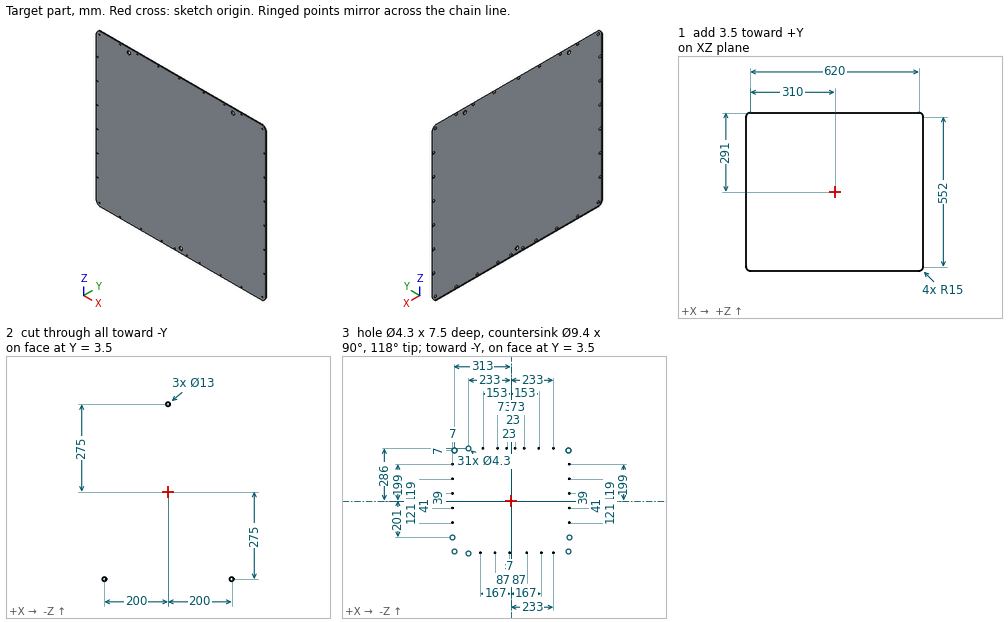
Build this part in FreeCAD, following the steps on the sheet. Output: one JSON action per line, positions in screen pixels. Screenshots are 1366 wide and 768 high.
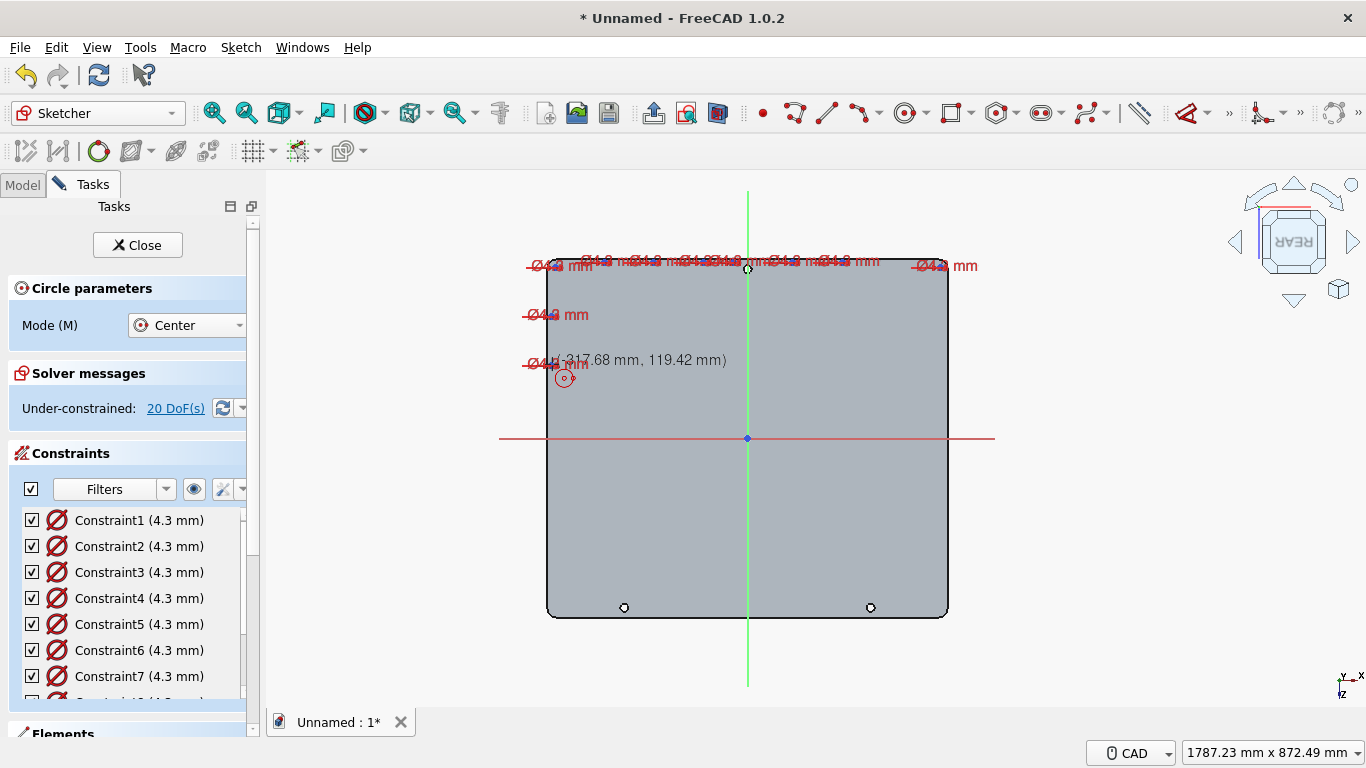
{"action": "scroll", "coordinate": [551, 414], "scroll_direction": "up", "scroll_amount": 15}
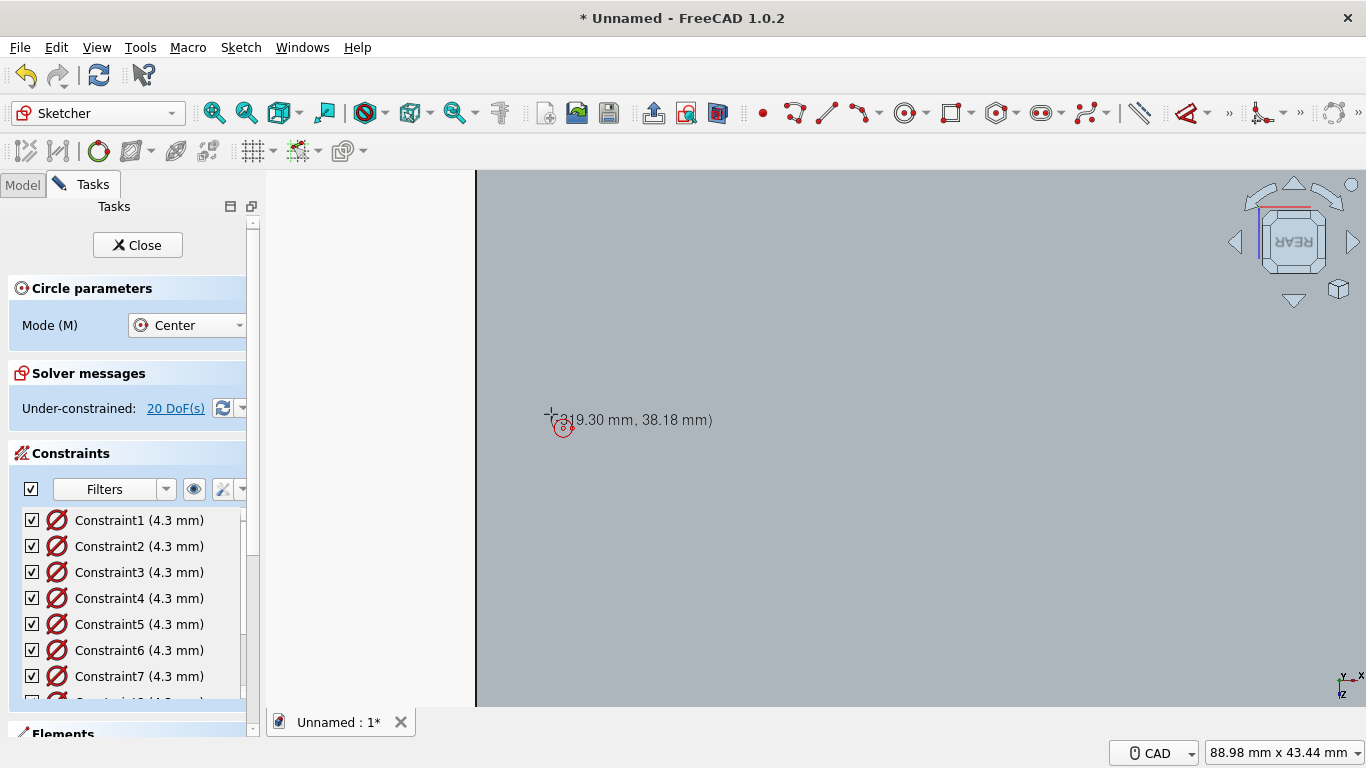
{"action": "scroll", "coordinate": [551, 414], "scroll_direction": "down", "scroll_amount": 15}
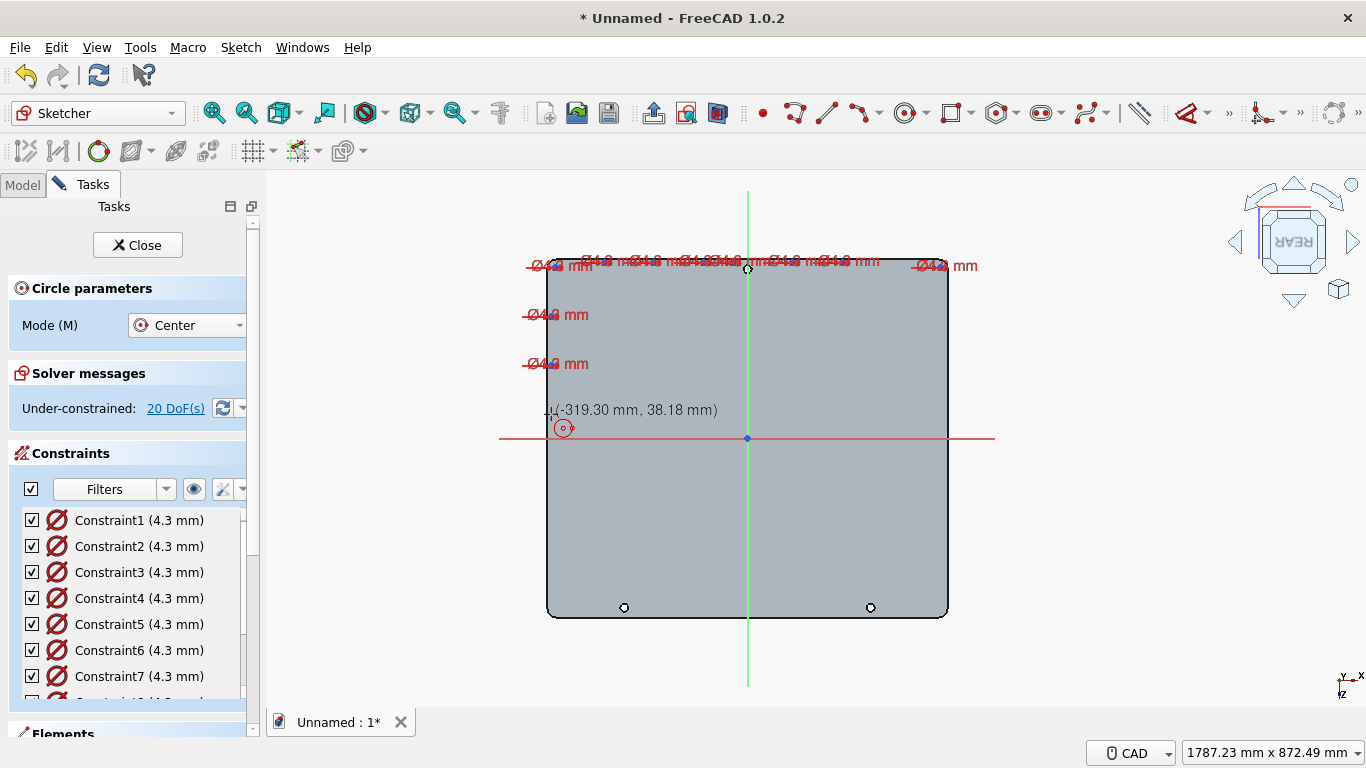
{"action": "left_click", "coordinate": [551, 414]}
{"action": "mouse_move", "coordinate": [552, 414]}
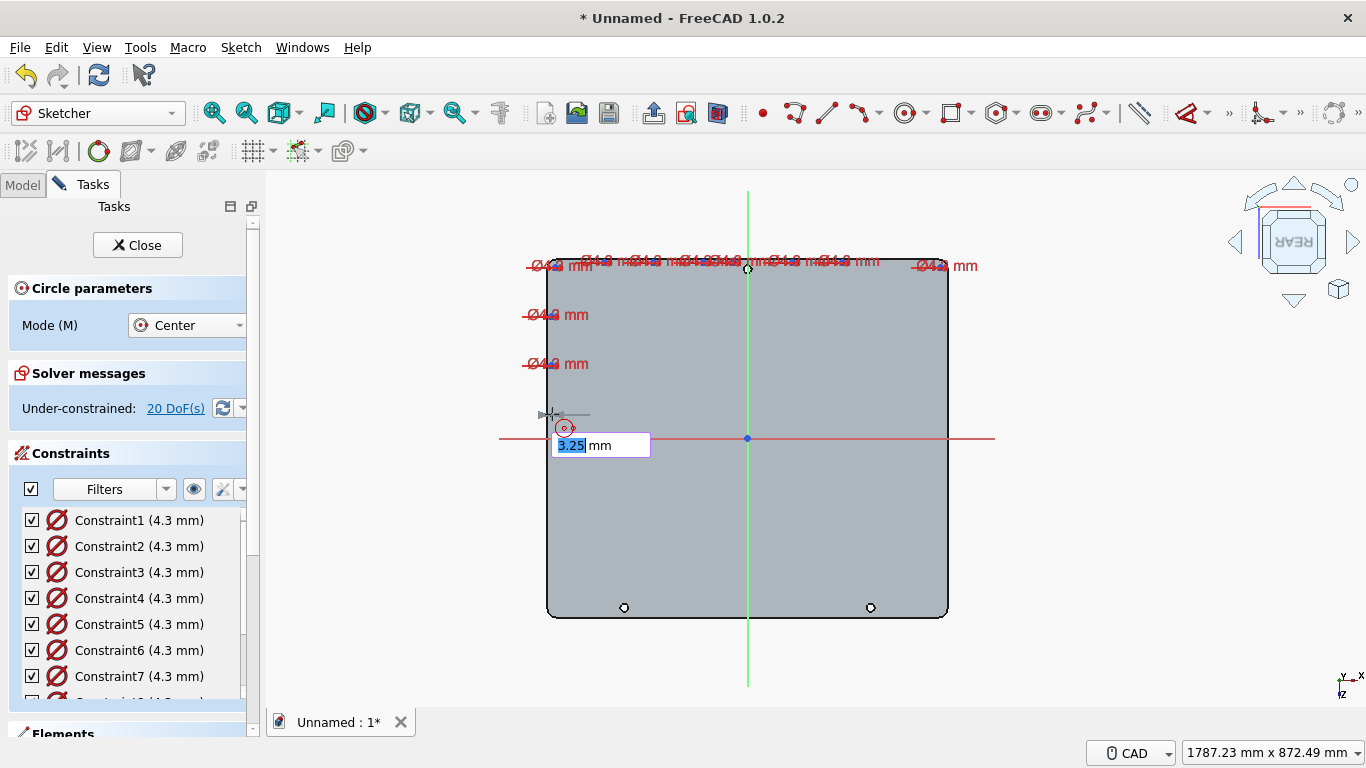
{"action": "type", "text": "4.3"}
{"action": "key", "text": "Return"}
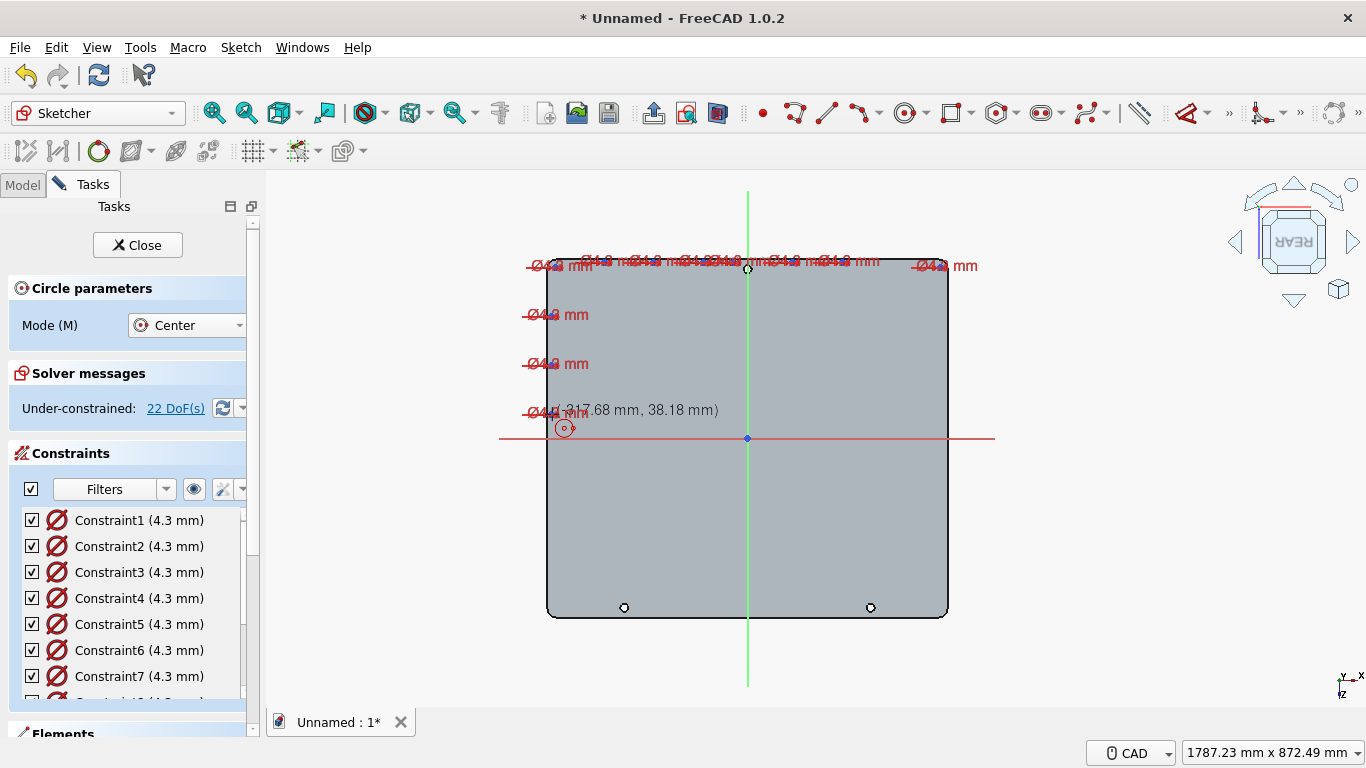
{"action": "scroll", "coordinate": [551, 464], "scroll_direction": "up", "scroll_amount": 15}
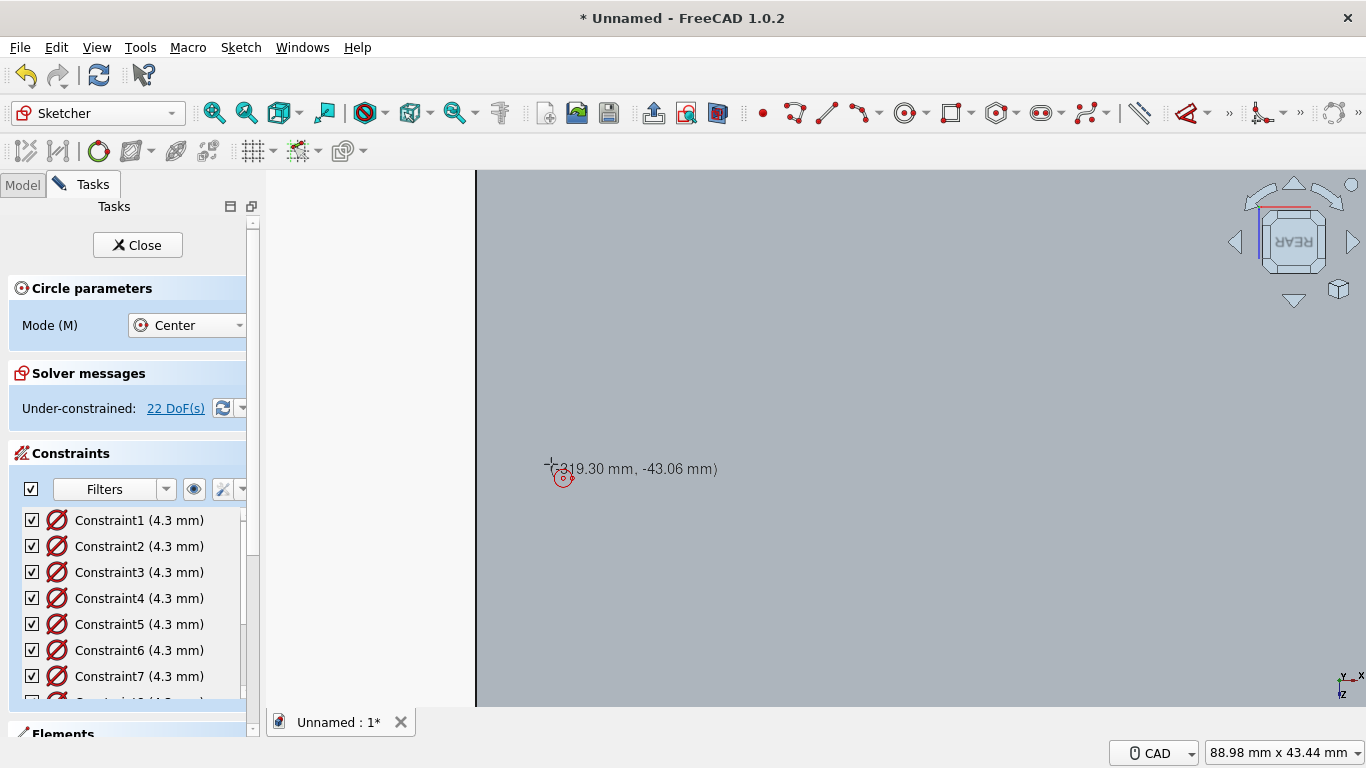
{"action": "scroll", "coordinate": [551, 465], "scroll_direction": "down", "scroll_amount": 15}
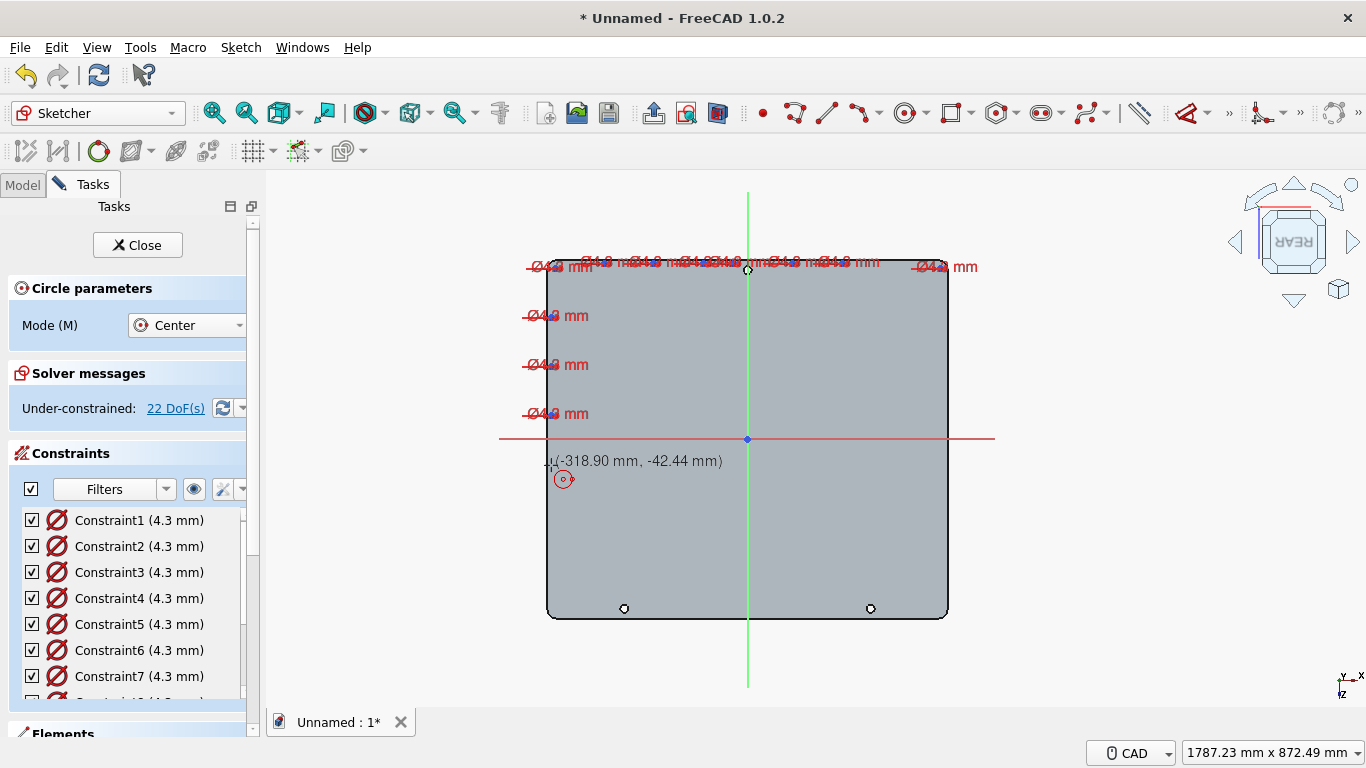
{"action": "left_click", "coordinate": [551, 465]}
{"action": "mouse_move", "coordinate": [552, 464]}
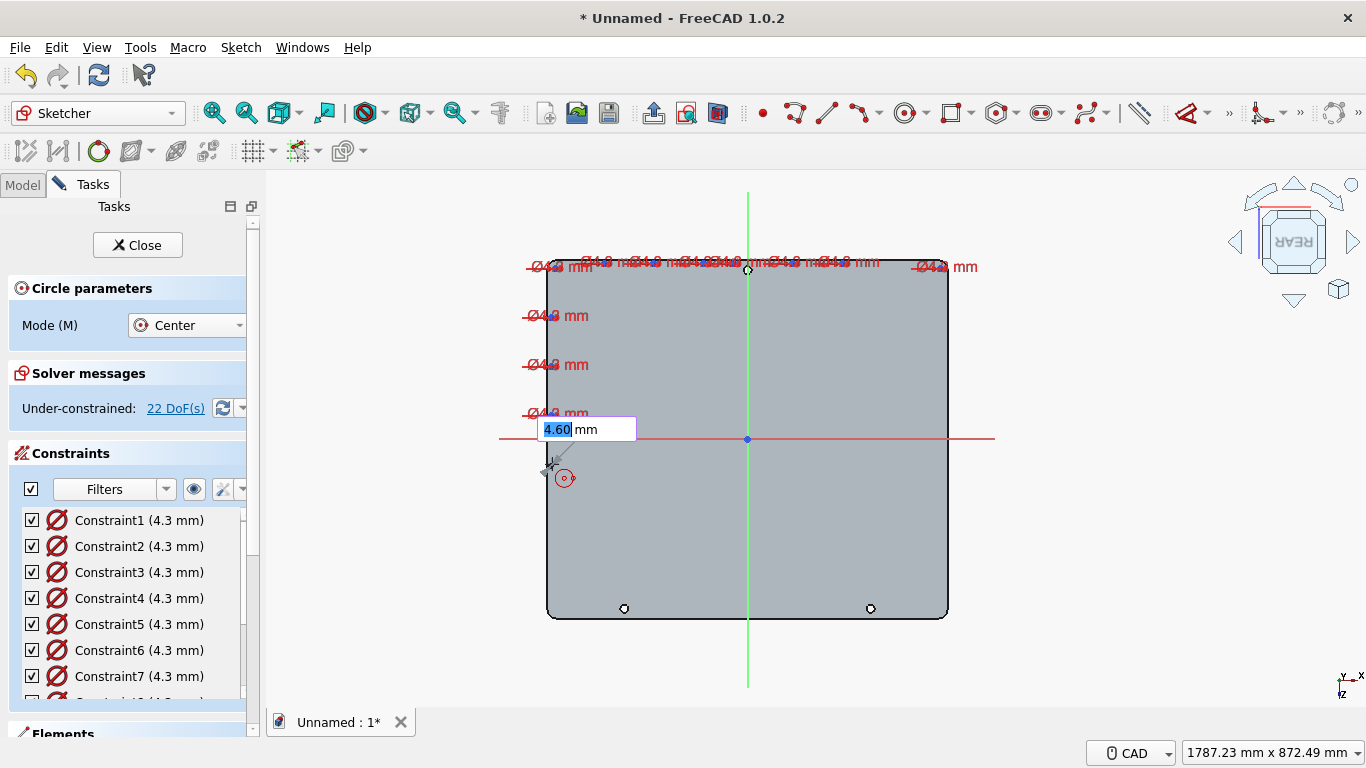
{"action": "type", "text": "4.3"}
{"action": "key", "text": "Return"}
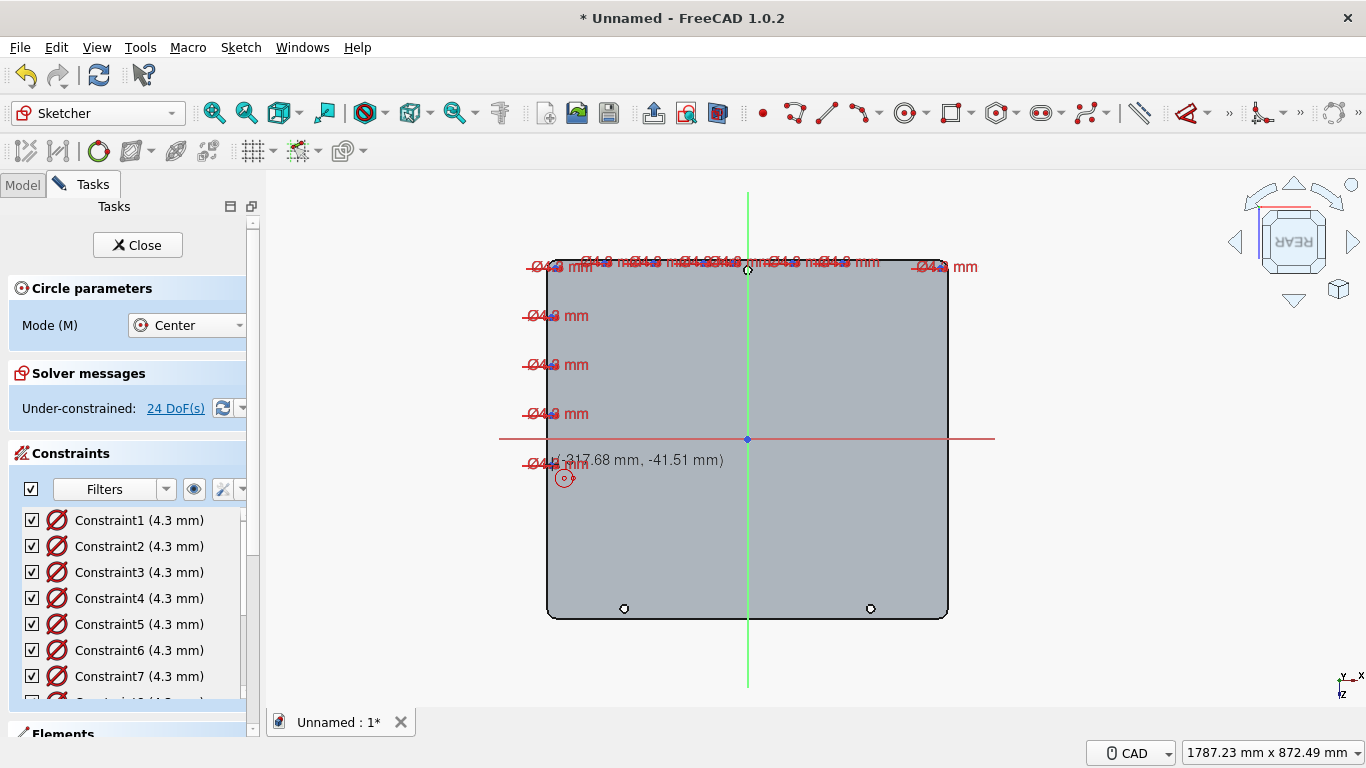
{"action": "scroll", "coordinate": [551, 514], "scroll_direction": "up", "scroll_amount": 15}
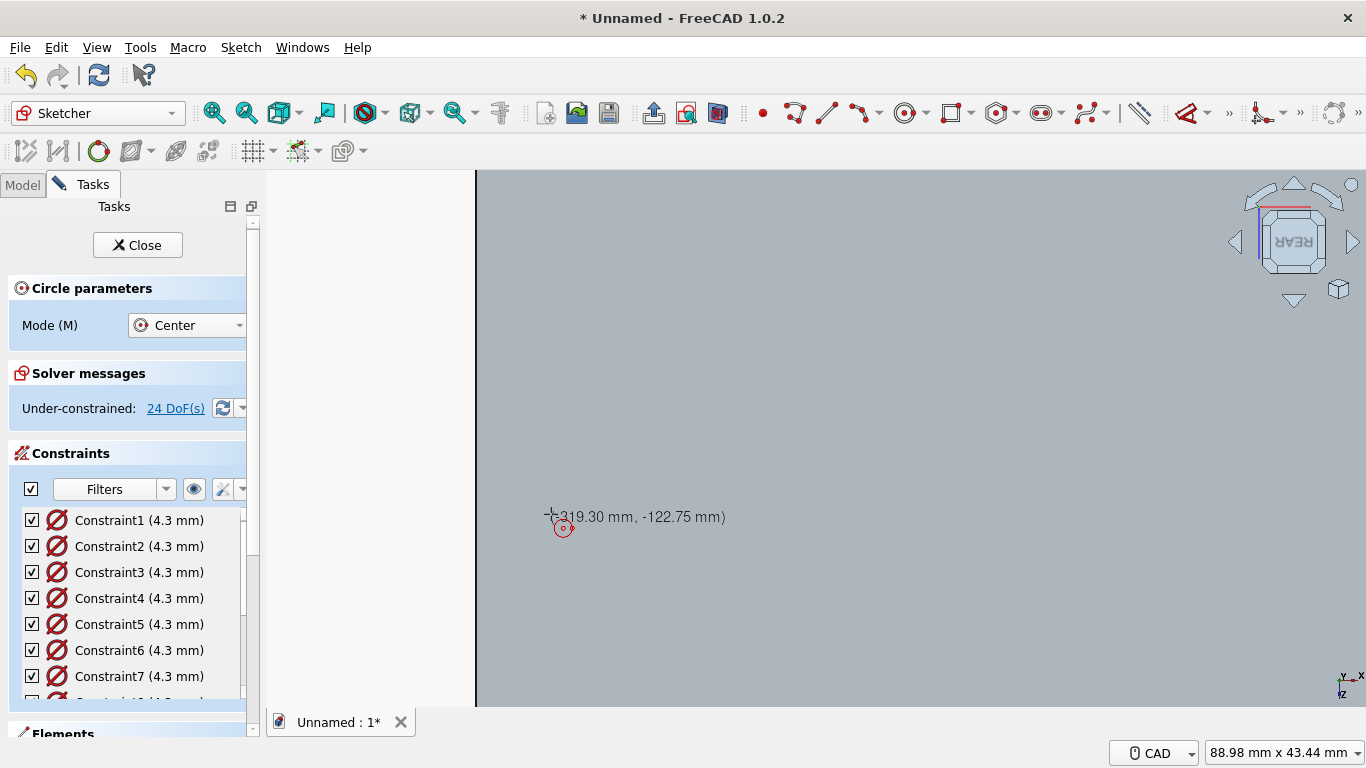
{"action": "scroll", "coordinate": [551, 514], "scroll_direction": "down", "scroll_amount": 15}